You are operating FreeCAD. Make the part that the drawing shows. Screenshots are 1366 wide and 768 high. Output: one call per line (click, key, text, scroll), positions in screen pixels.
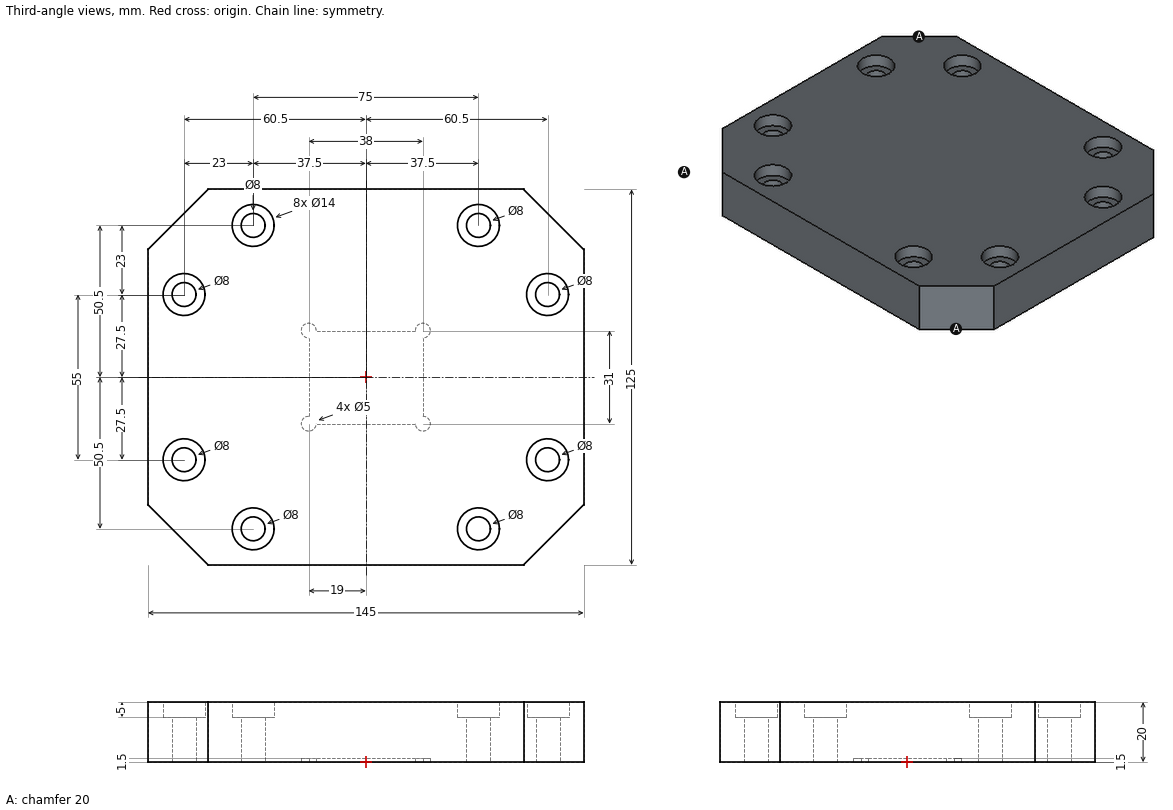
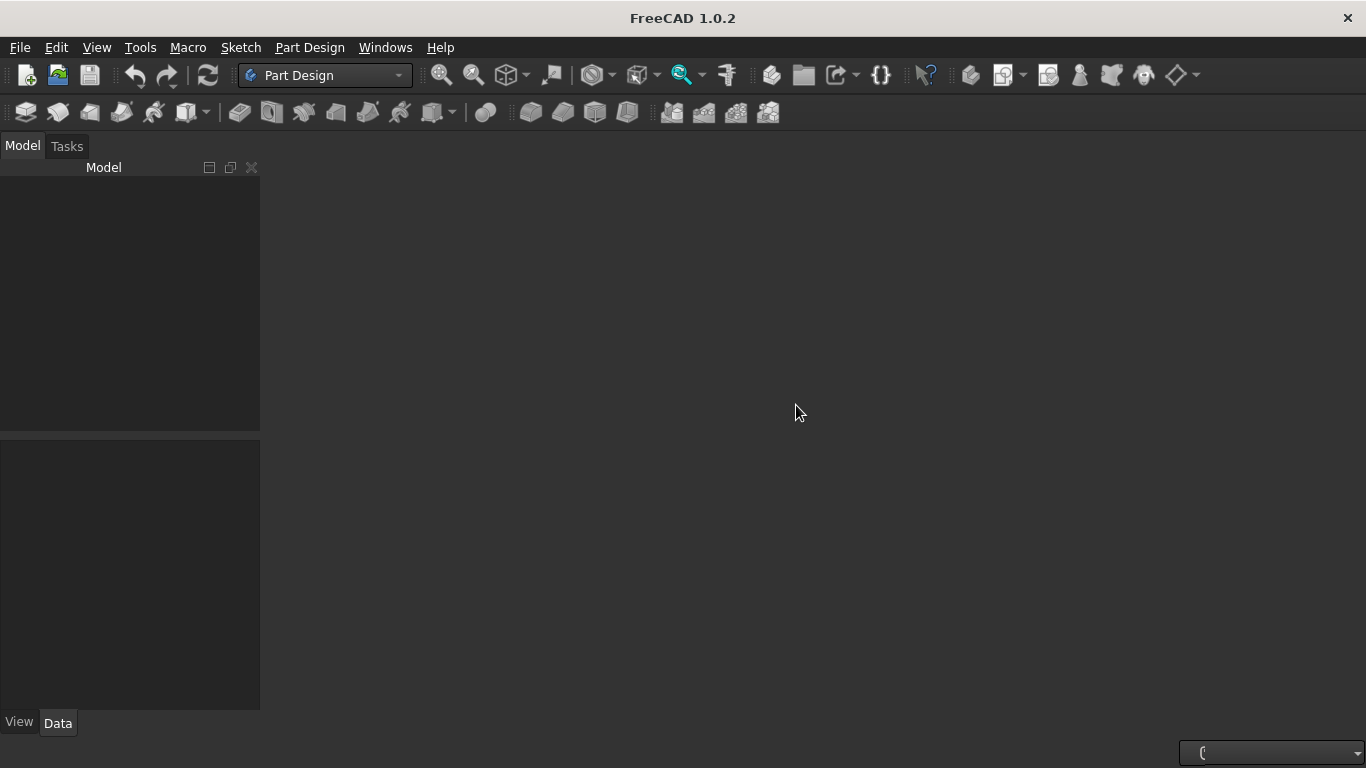
key(ctrl+n)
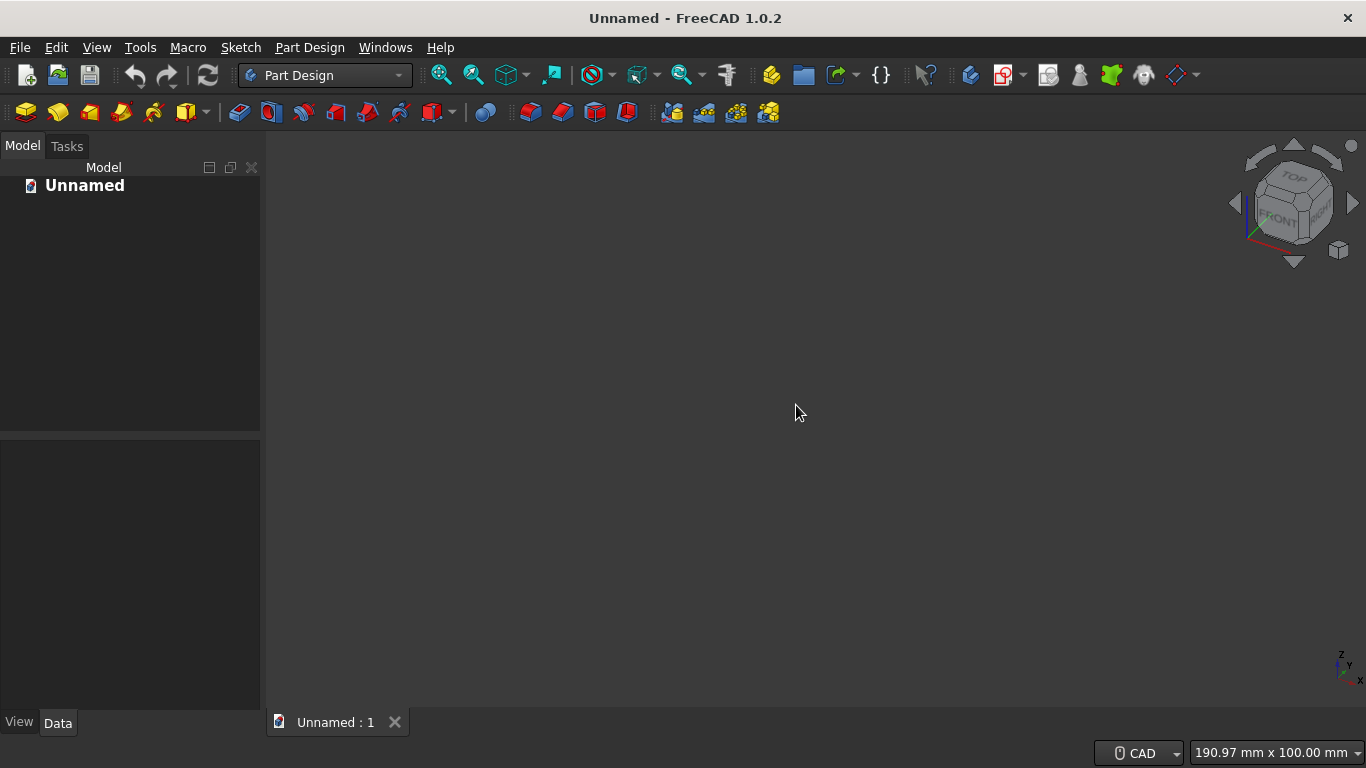
click(1004, 76)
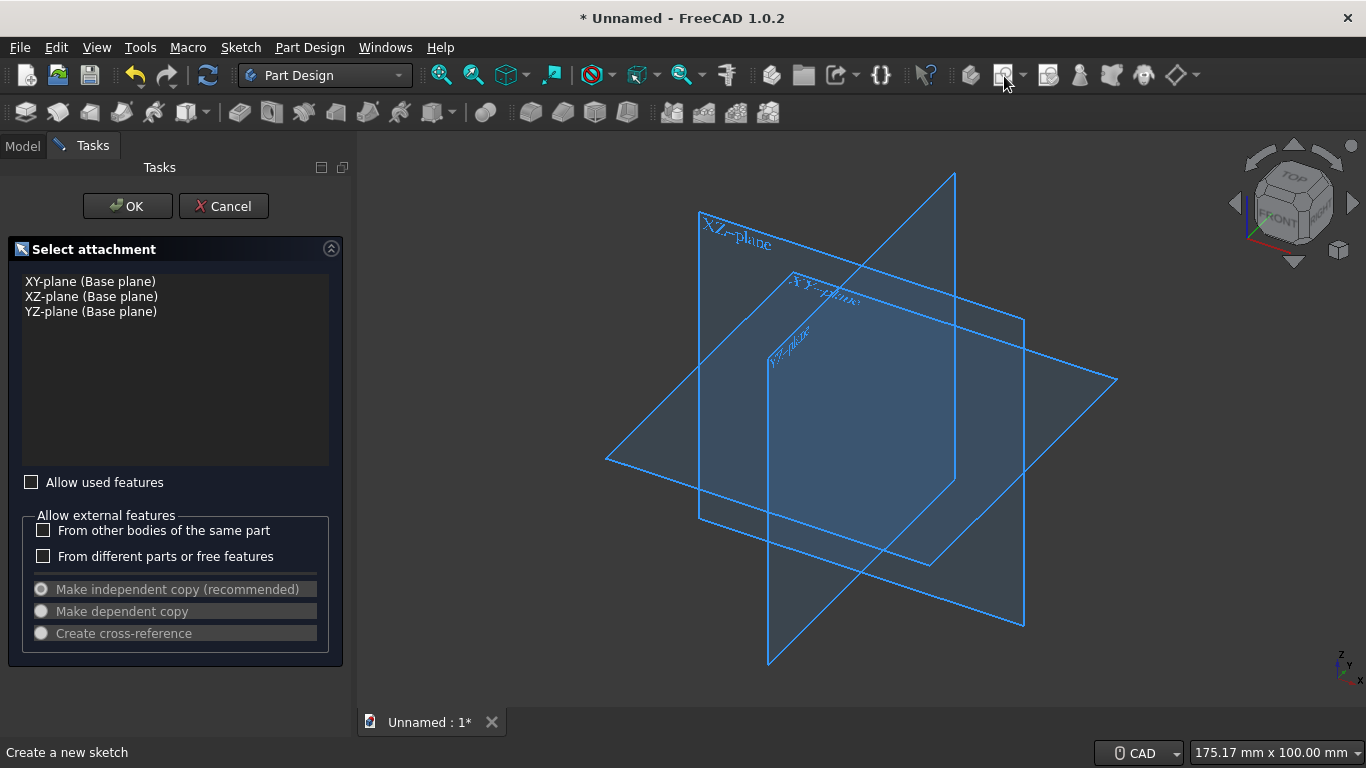
click(82, 282)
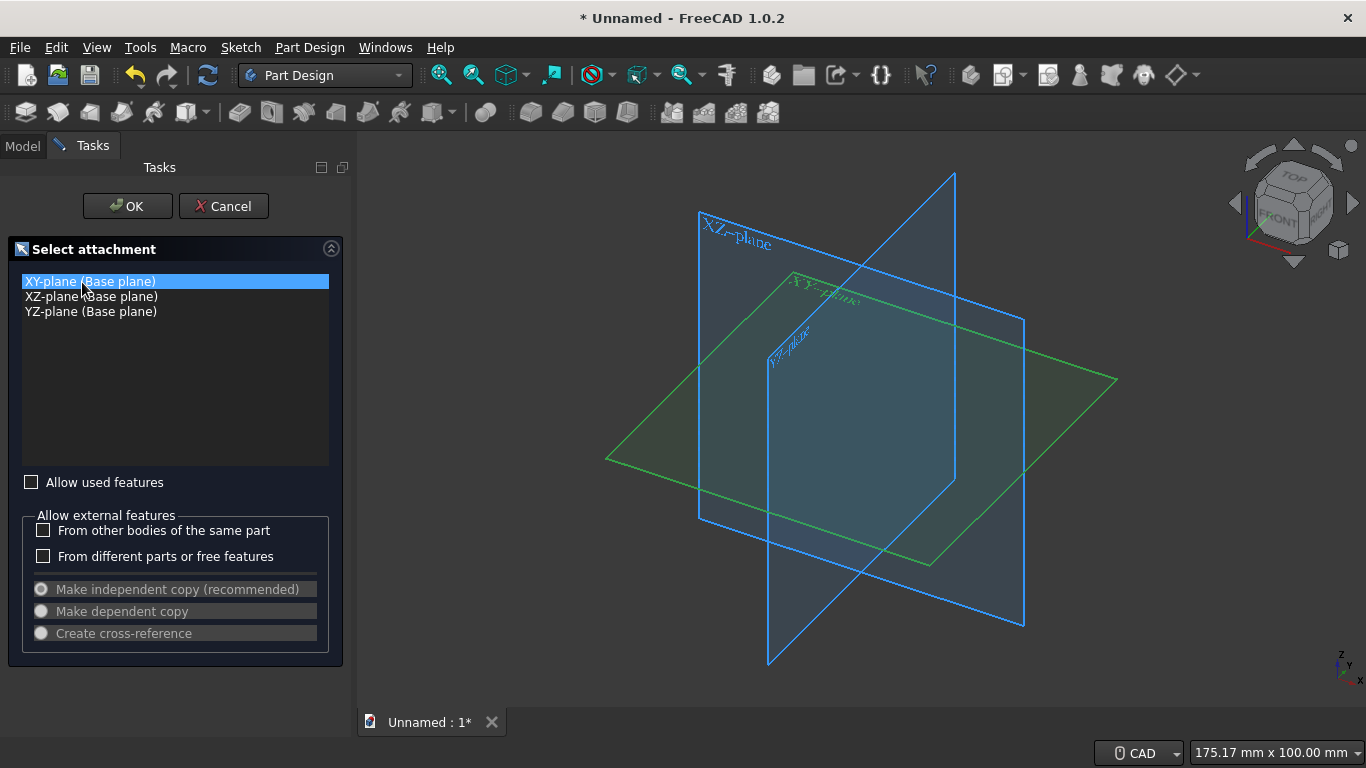
click(128, 206)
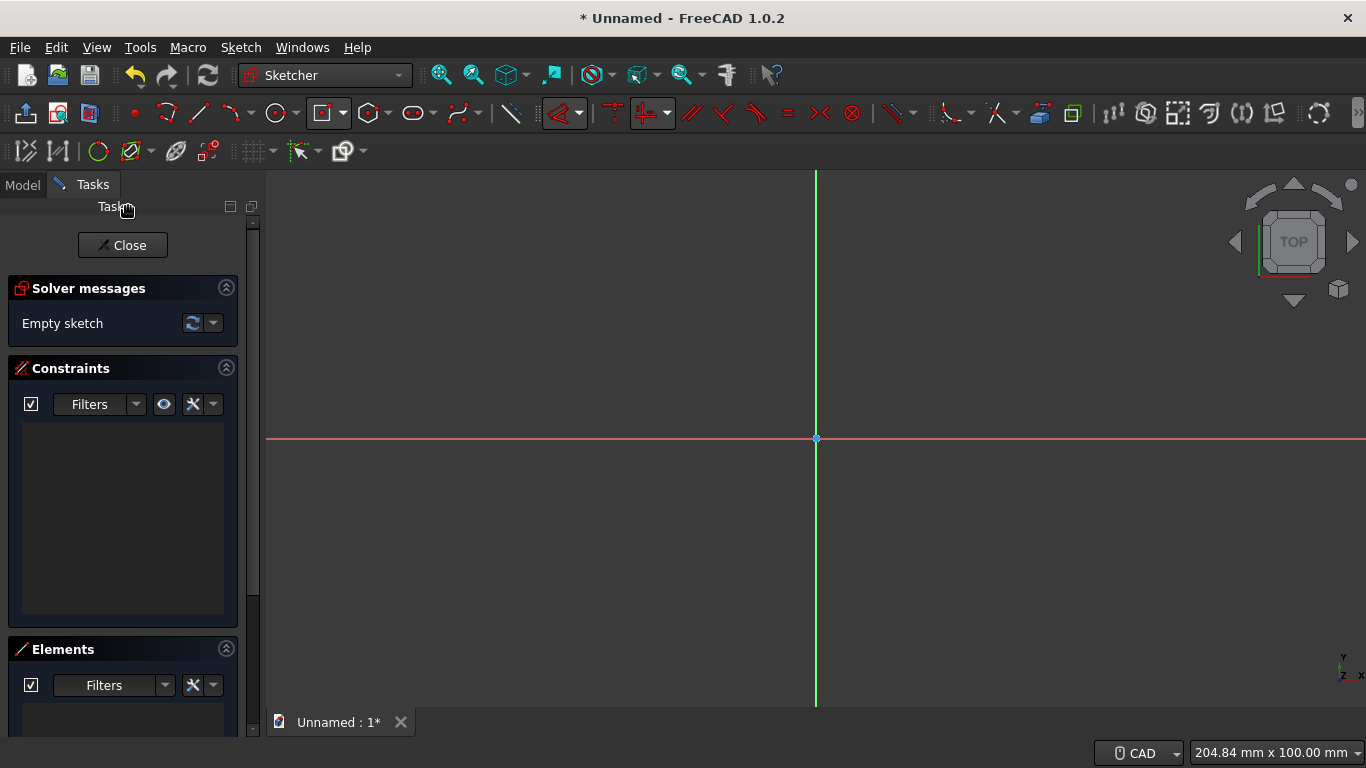
scroll(664, 438, down, 3)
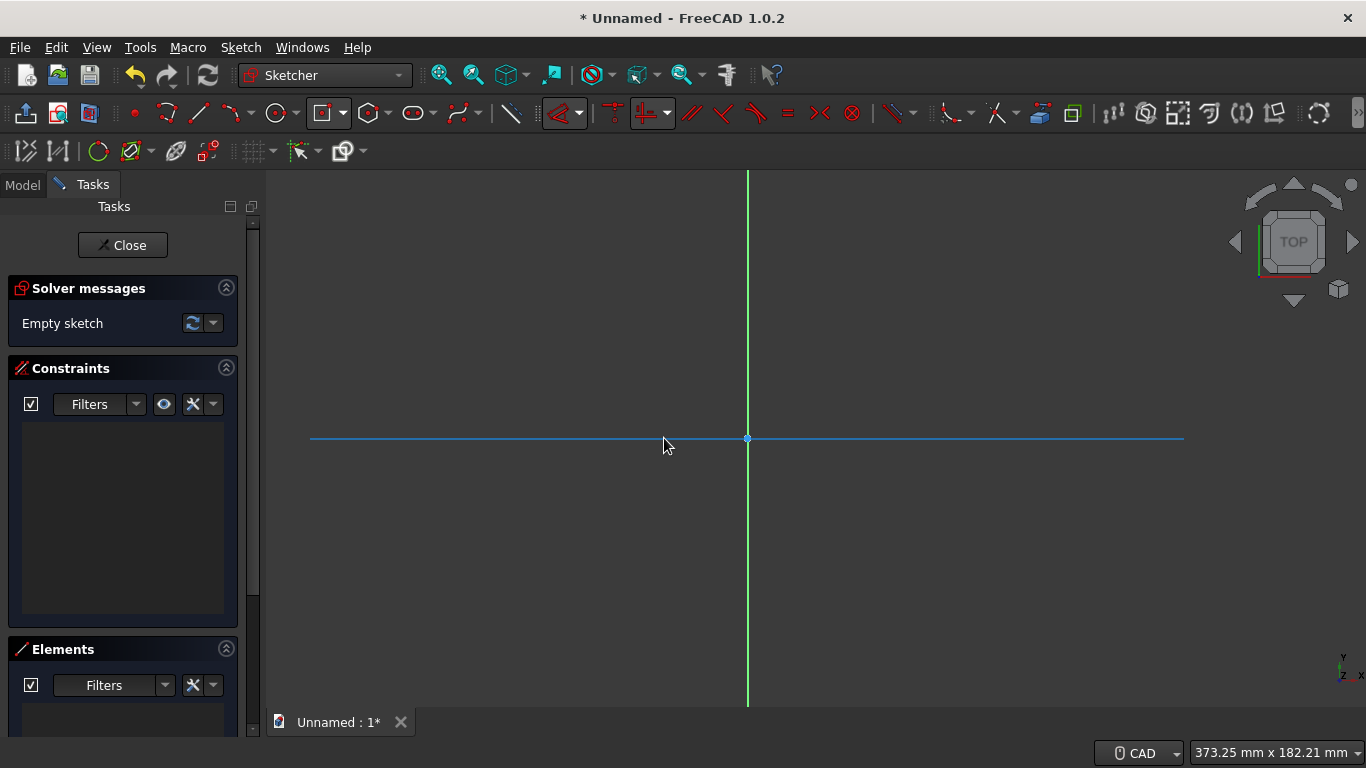
key(g)
key(v)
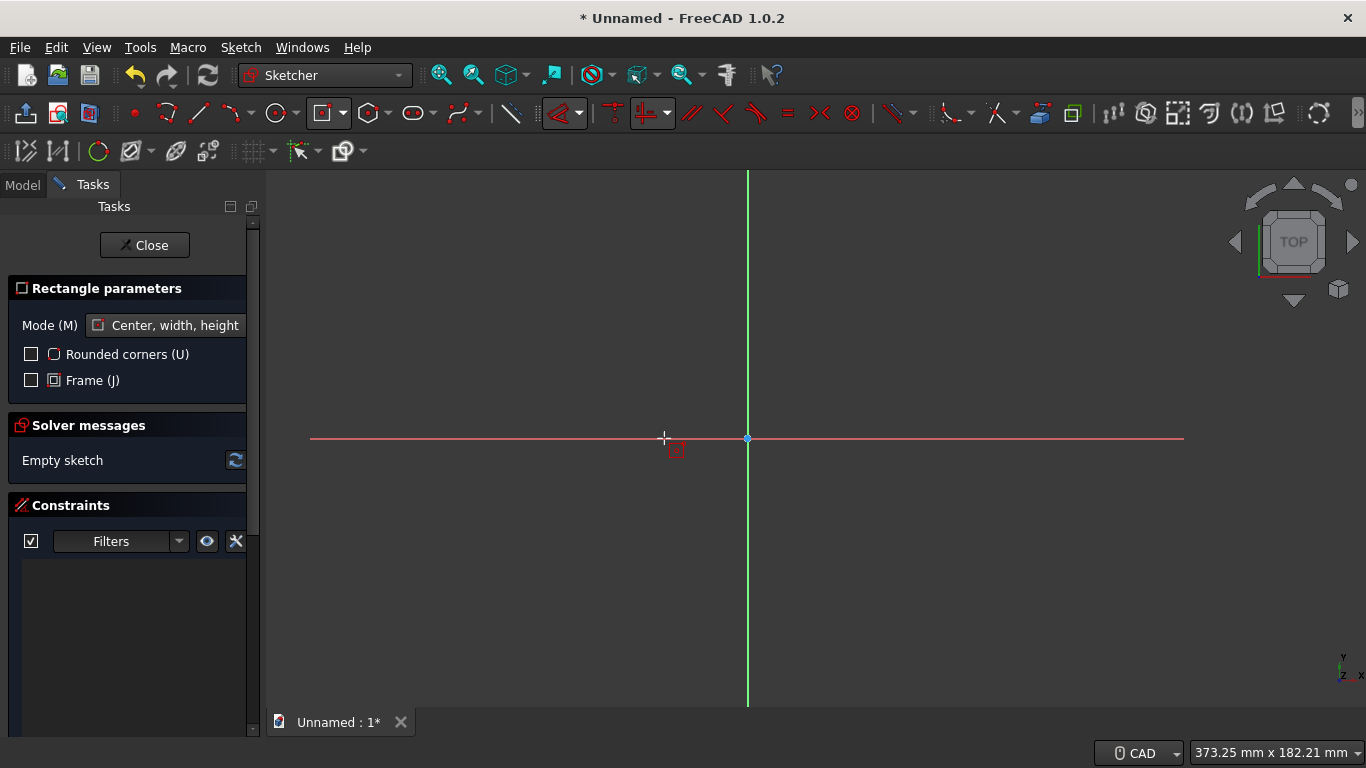
click(748, 438)
click(961, 254)
key(Escape)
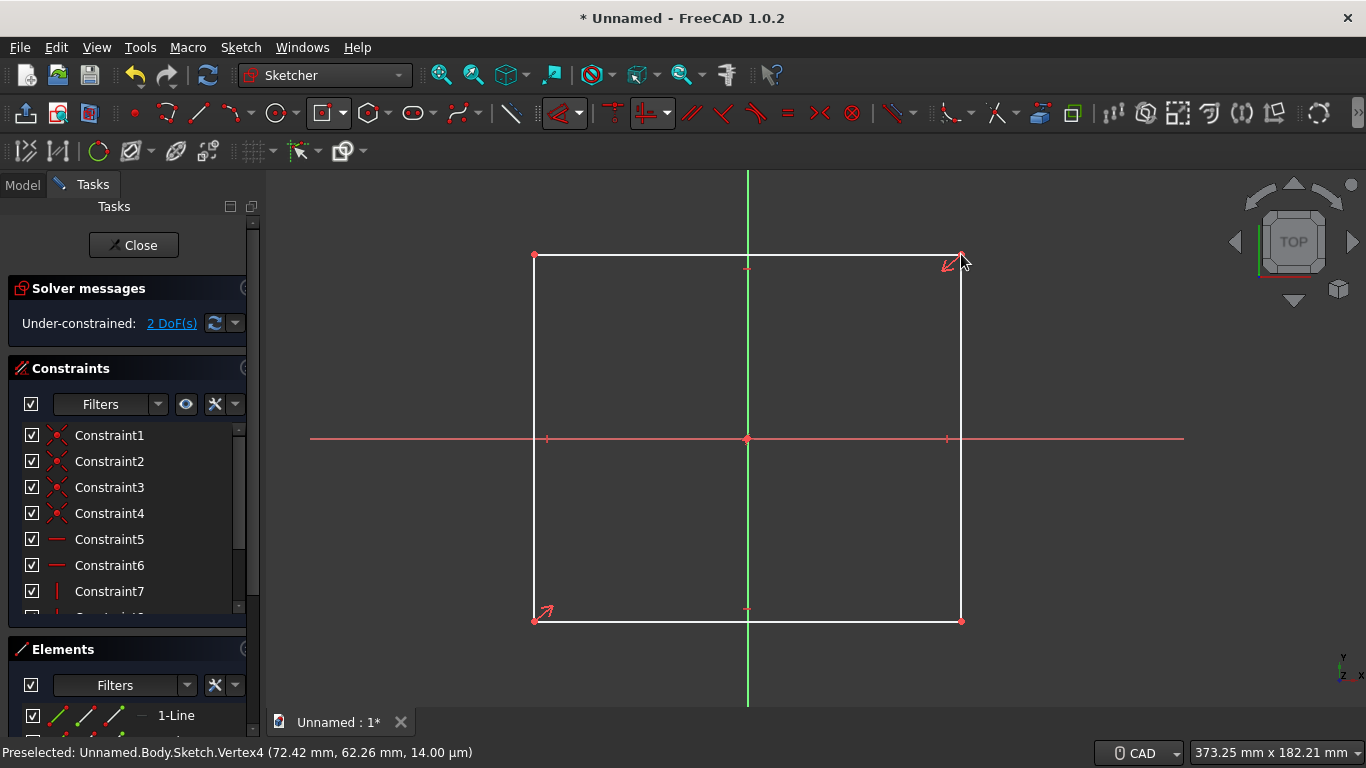
click(662, 622)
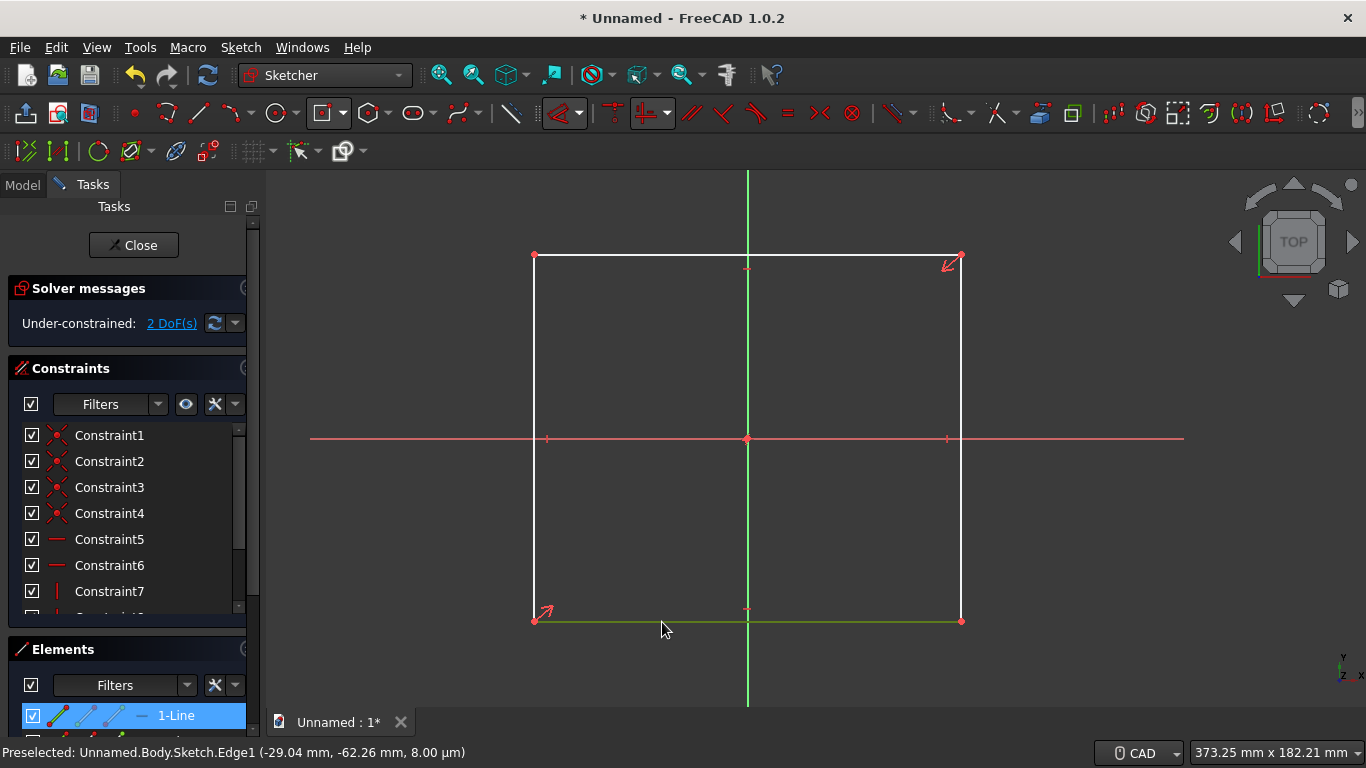
key(l)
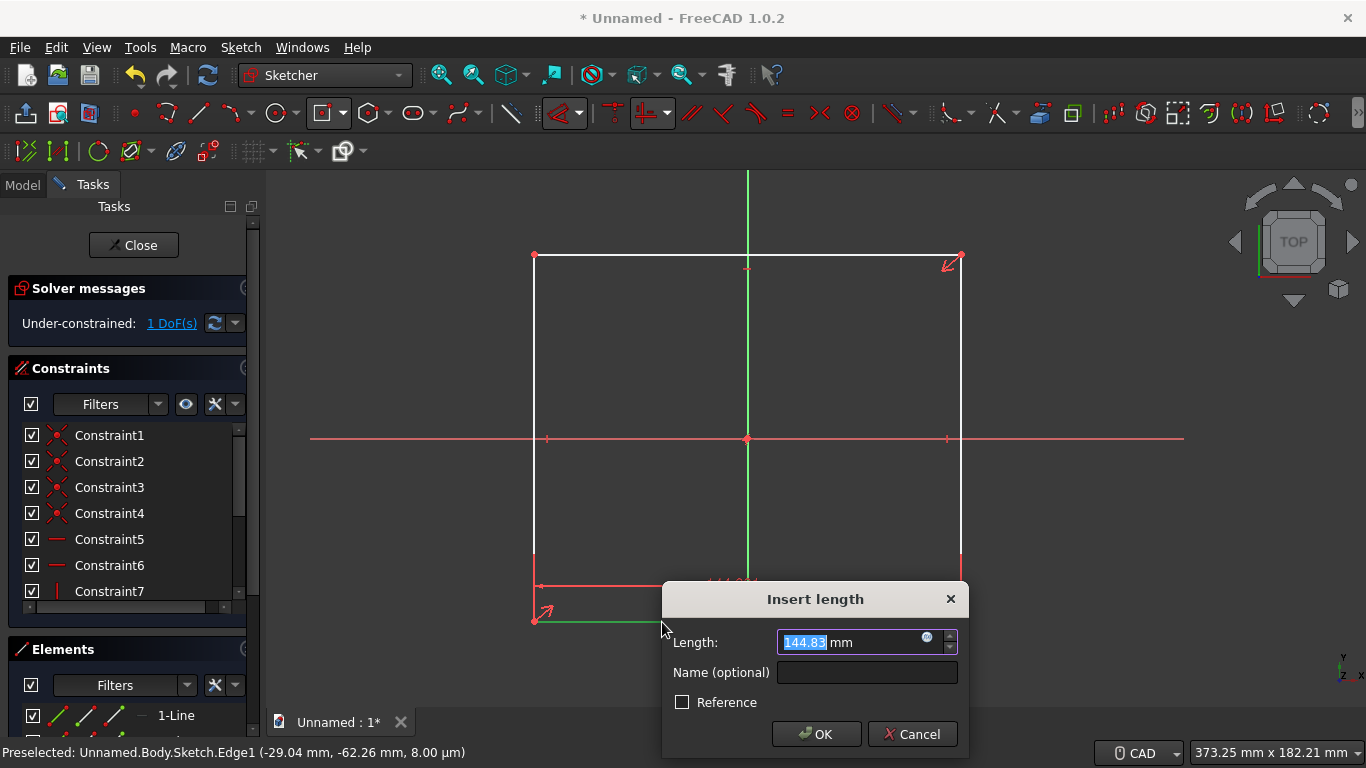
text(145)
key(Return)